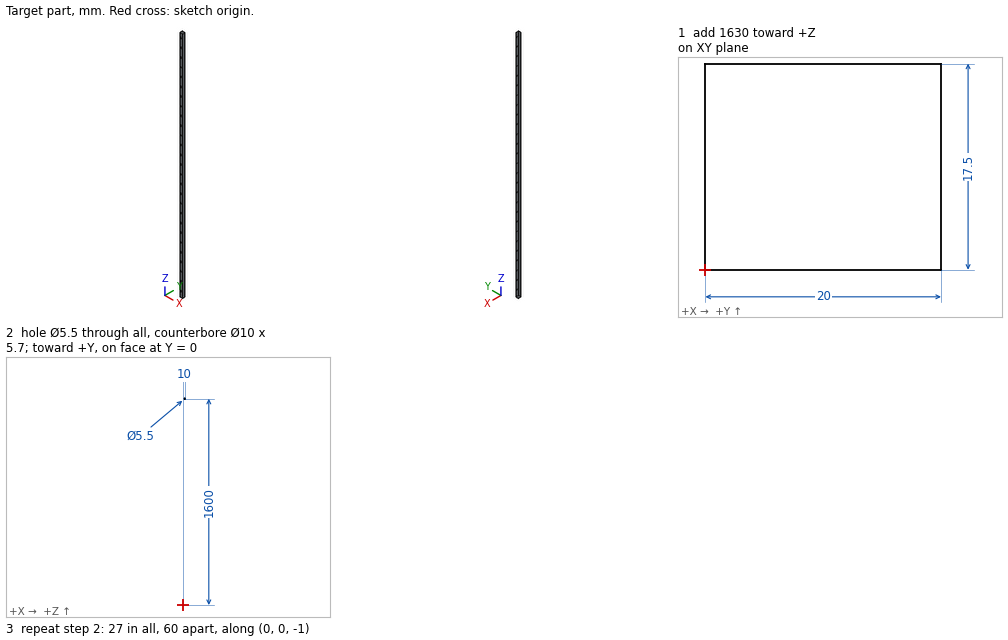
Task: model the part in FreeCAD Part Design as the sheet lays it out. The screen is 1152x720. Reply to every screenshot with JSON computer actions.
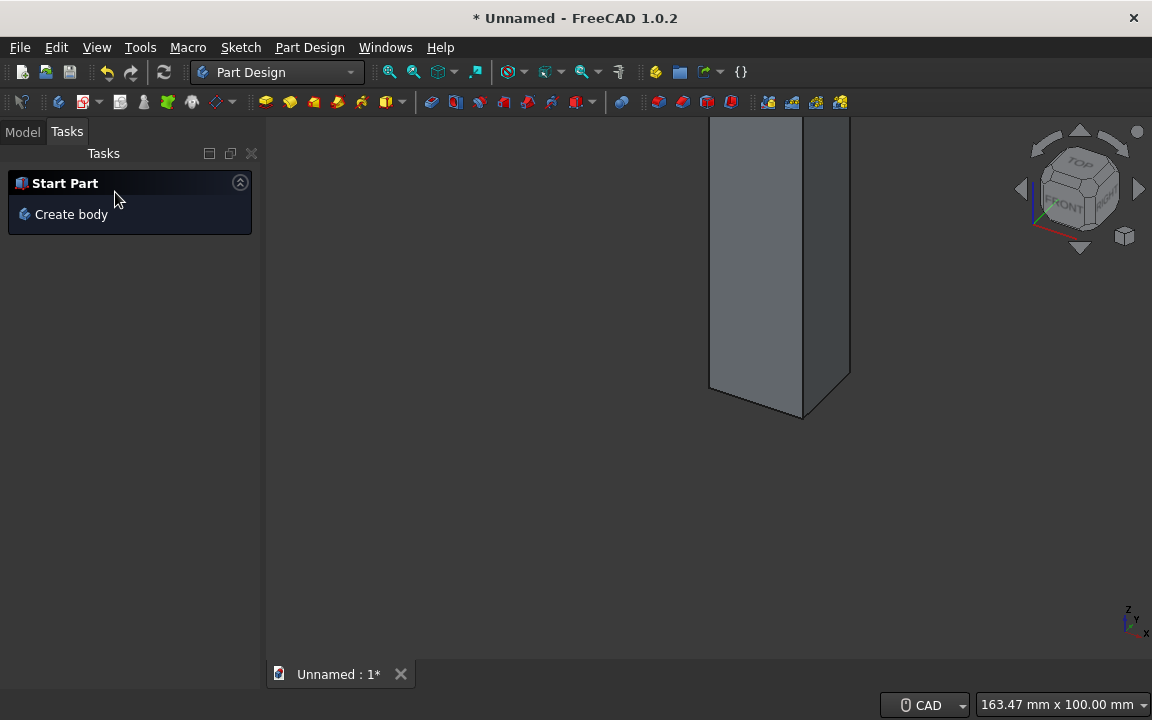
{"action": "left_click", "coordinate": [390, 72]}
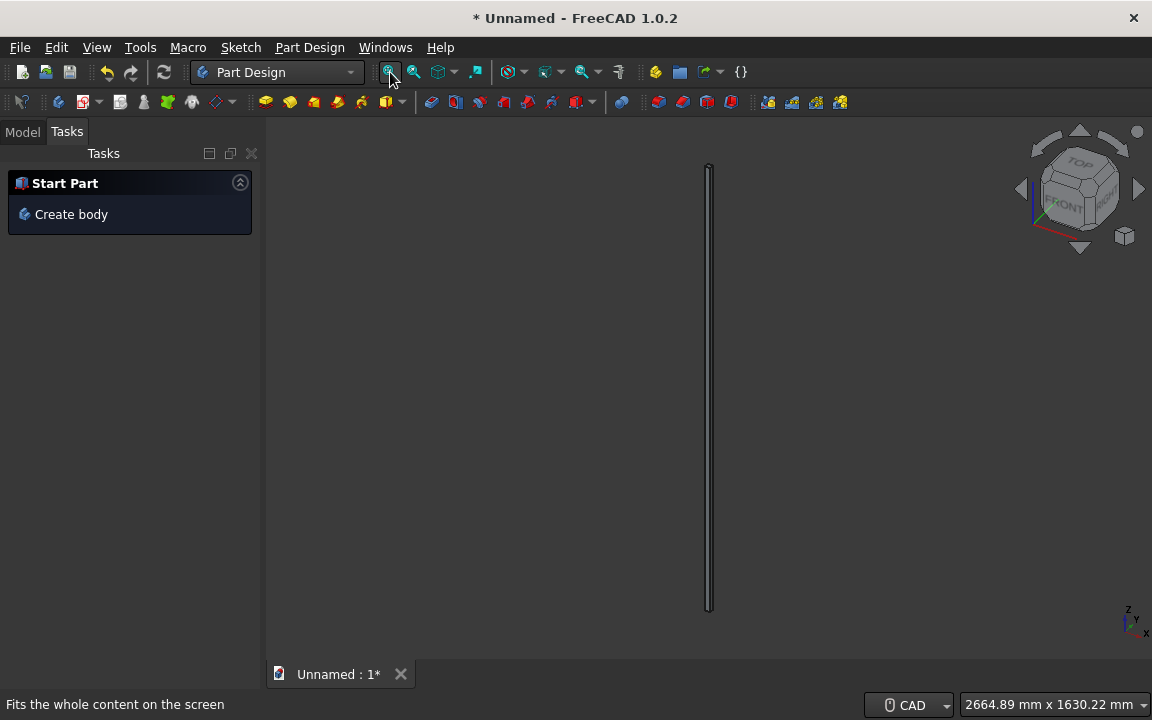
{"action": "scroll", "coordinate": [708, 198], "scroll_direction": "up", "scroll_amount": 7}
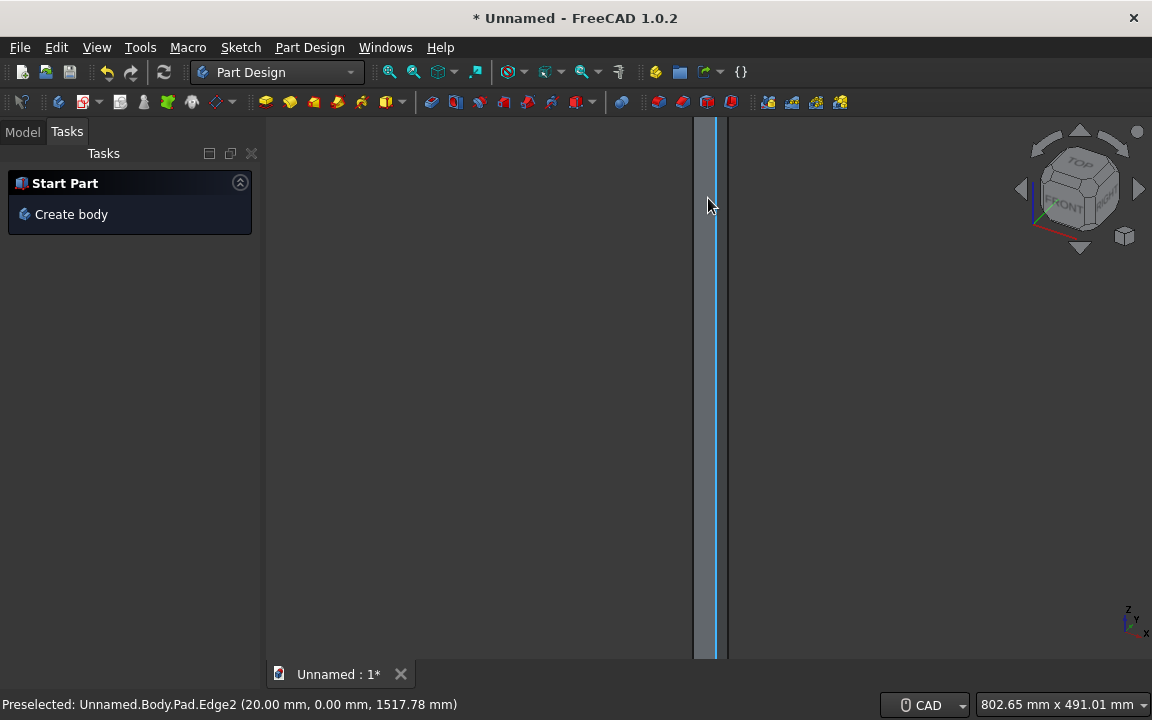
{"action": "left_click", "coordinate": [705, 201]}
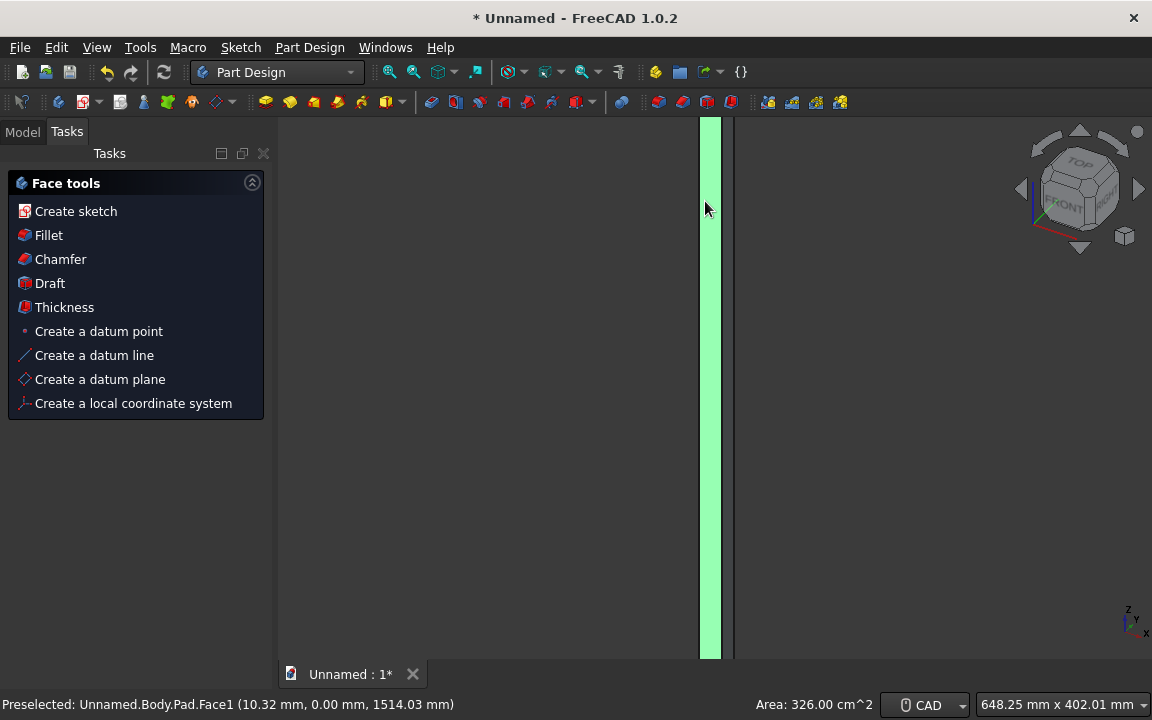
{"action": "left_click", "coordinate": [84, 102]}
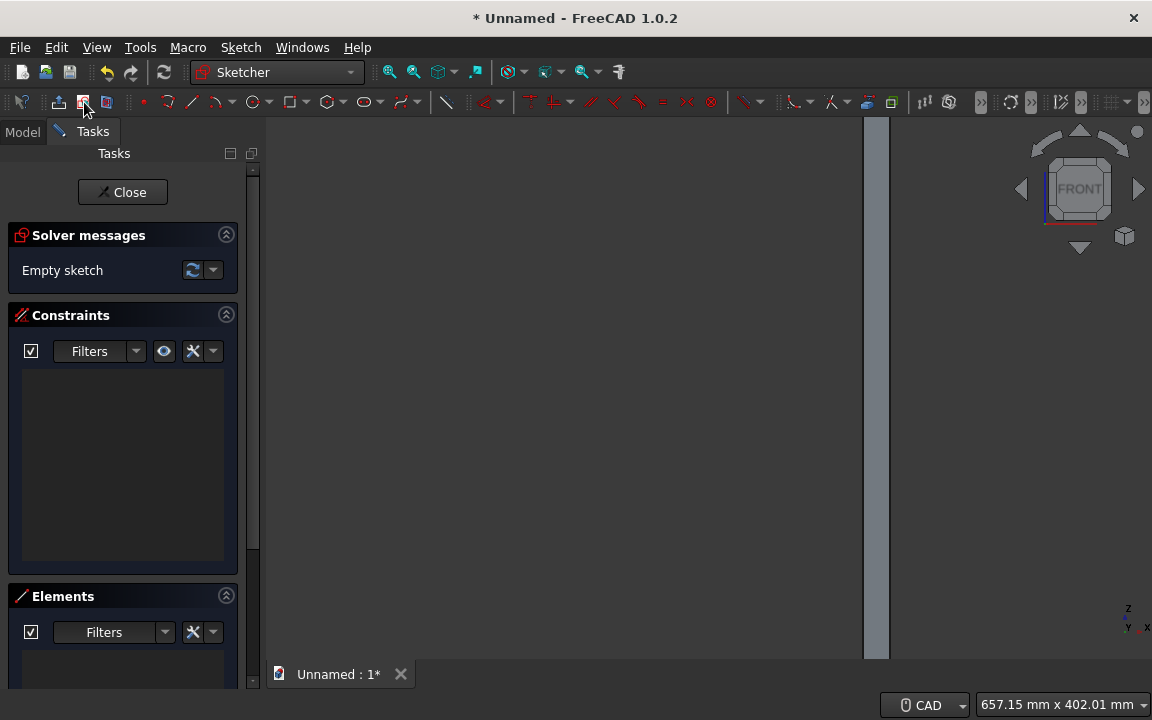
{"action": "scroll", "coordinate": [640, 388], "scroll_direction": "down", "scroll_amount": 5}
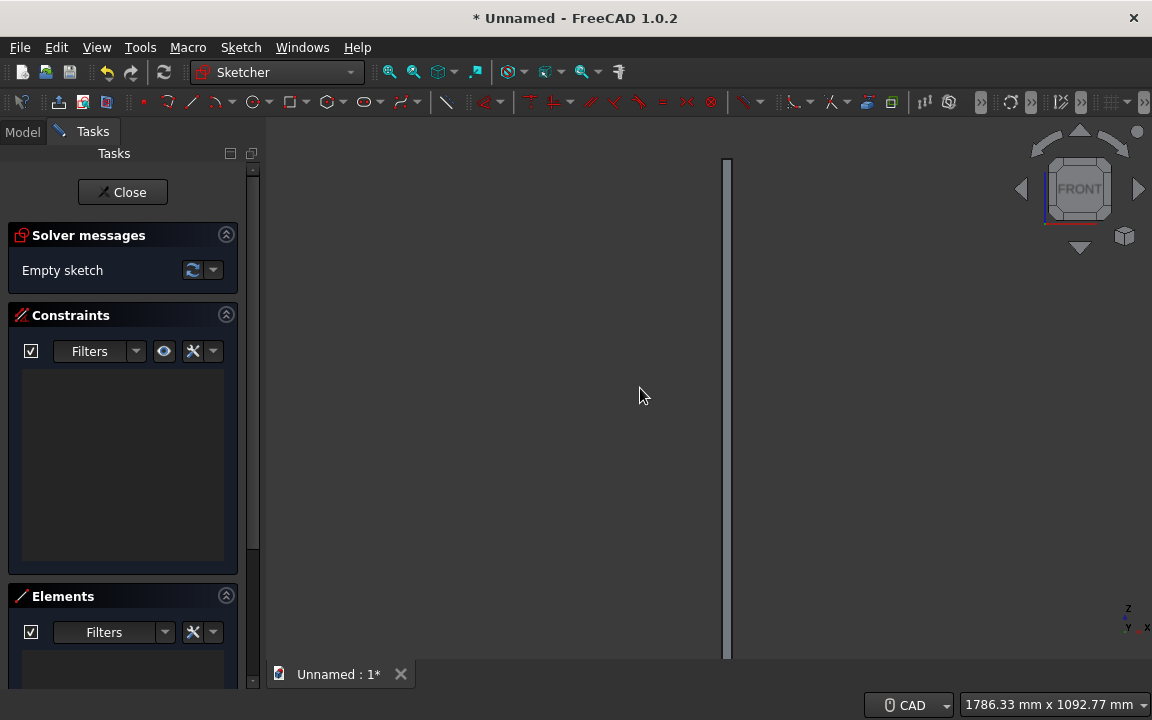
{"action": "scroll", "coordinate": [732, 163], "scroll_direction": "up", "scroll_amount": 15}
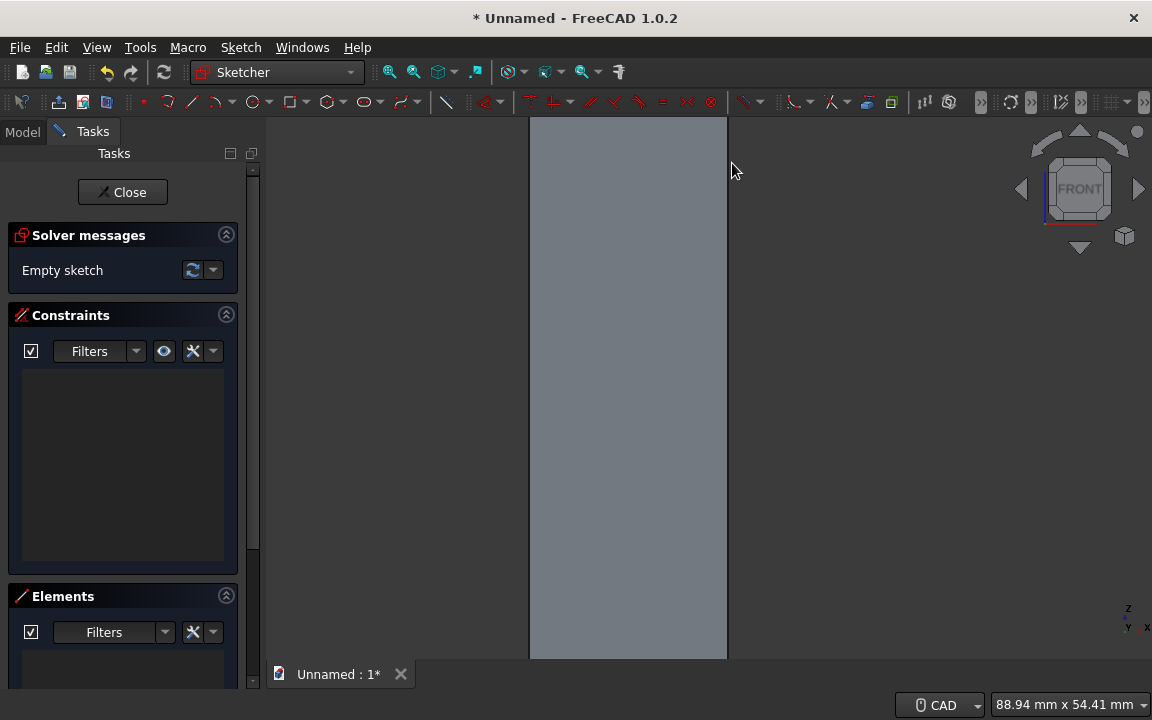
{"action": "scroll", "coordinate": [626, 375], "scroll_direction": "up", "scroll_amount": 9}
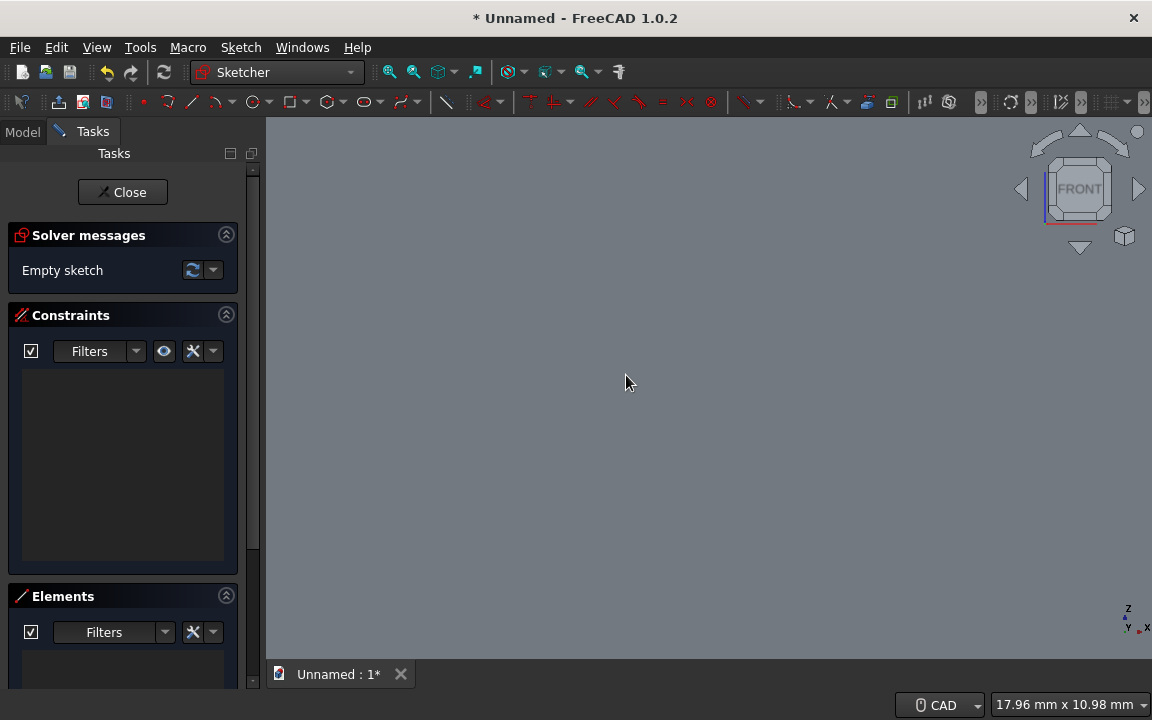
{"action": "left_click", "coordinate": [254, 102]}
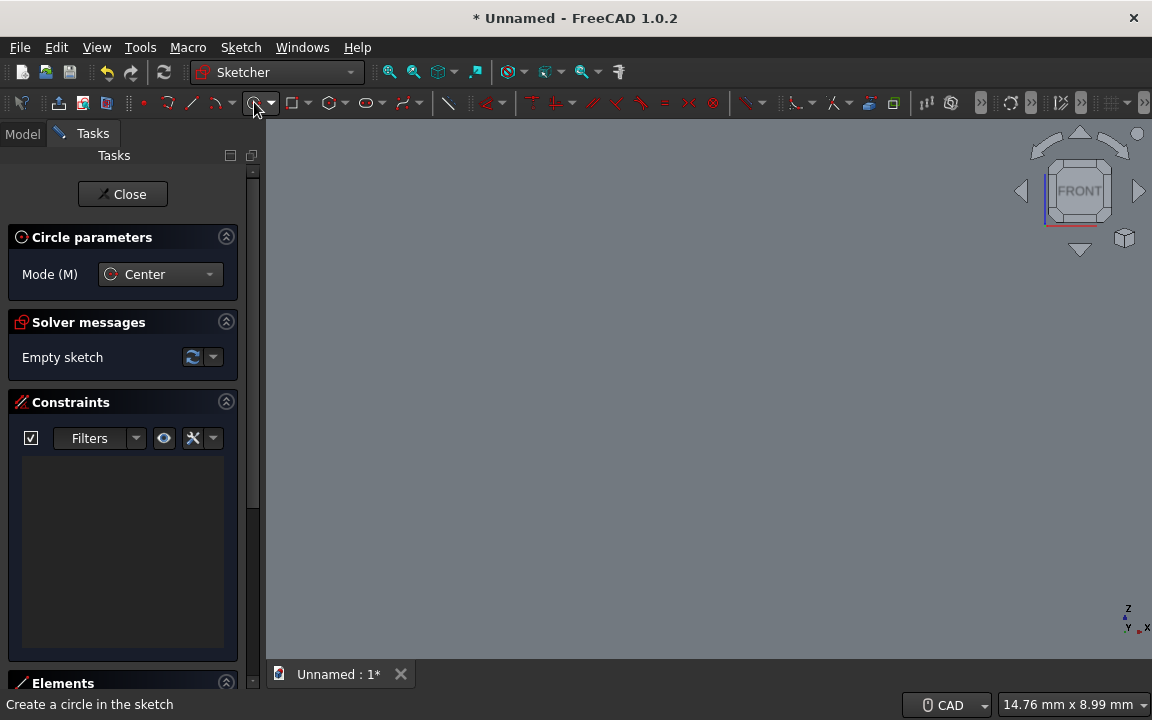
{"action": "left_click", "coordinate": [638, 388]}
{"action": "mouse_move", "coordinate": [754, 272]}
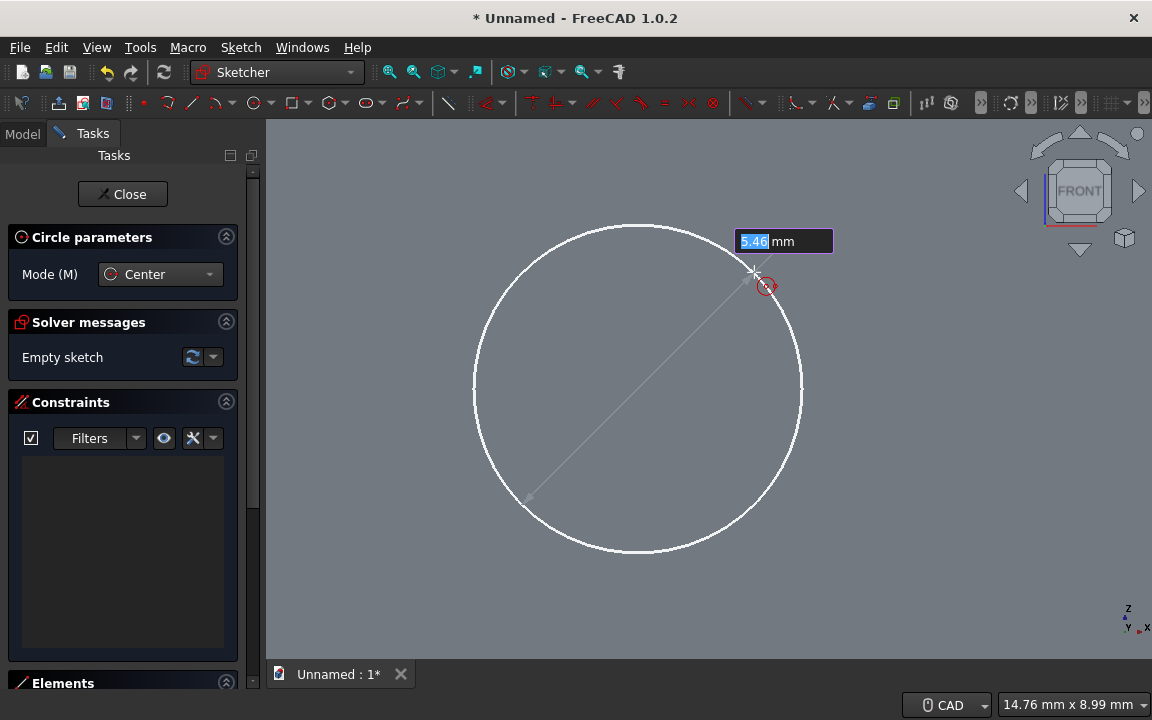
{"action": "type", "text": "5.5"}
{"action": "key", "text": "Return"}
{"action": "key", "text": "Escape"}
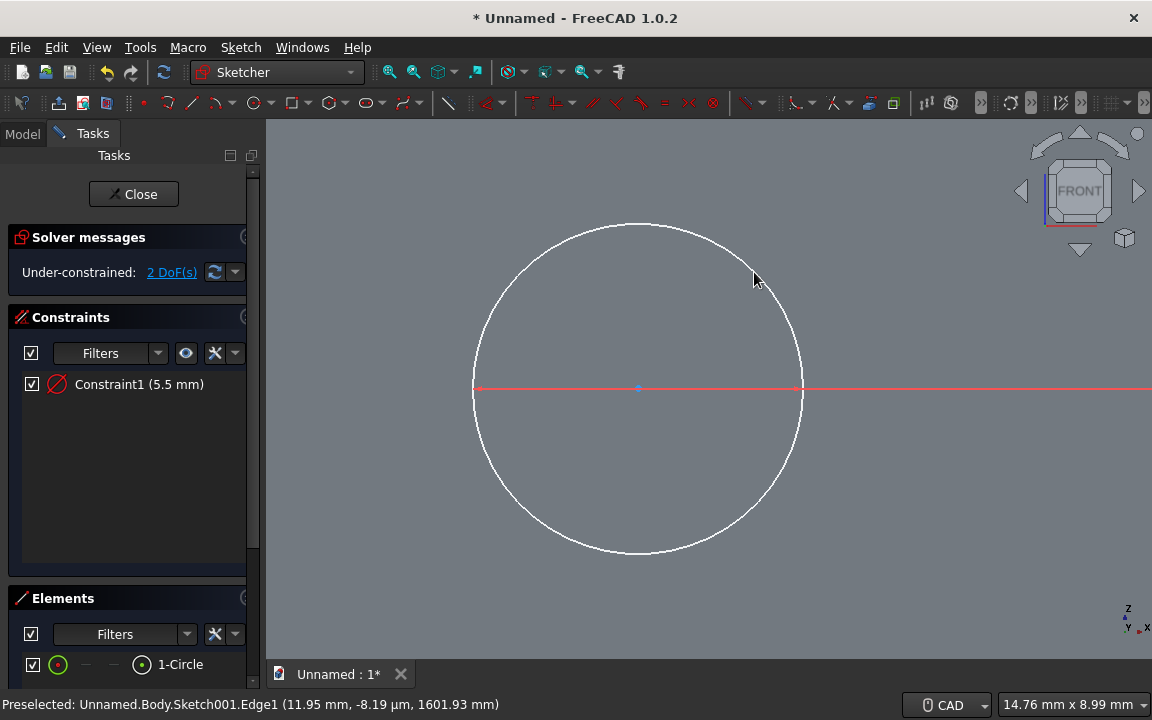
{"action": "left_click", "coordinate": [638, 389]}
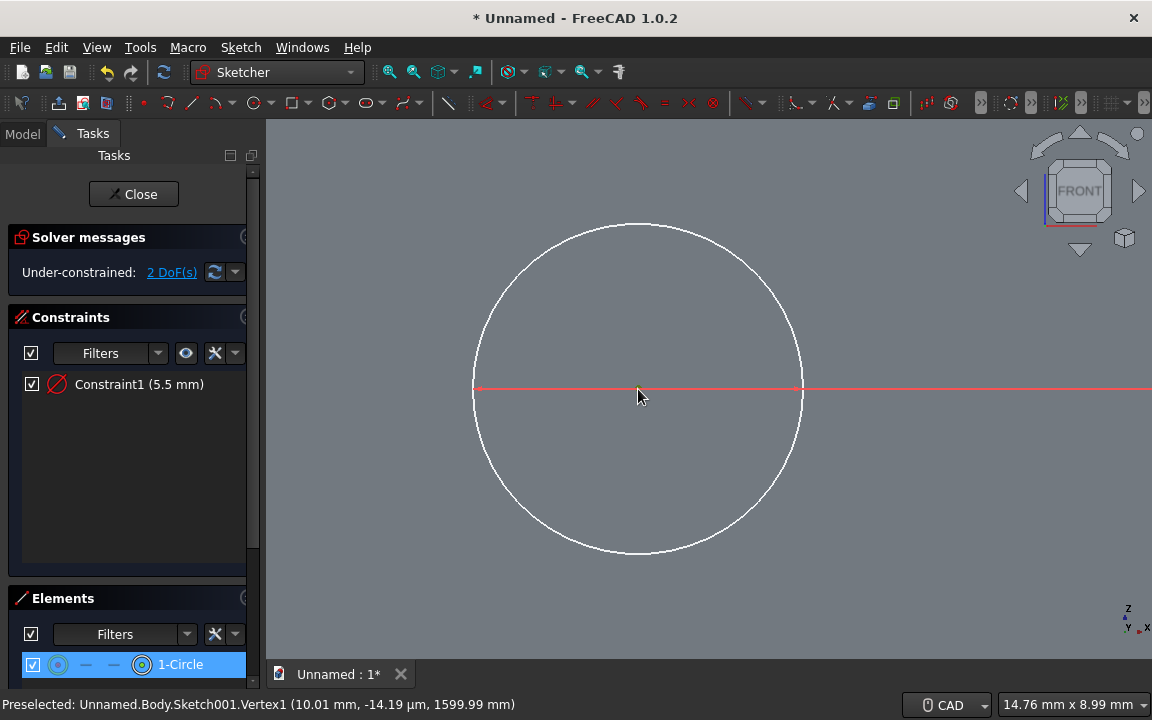
{"action": "key", "text": "l"}